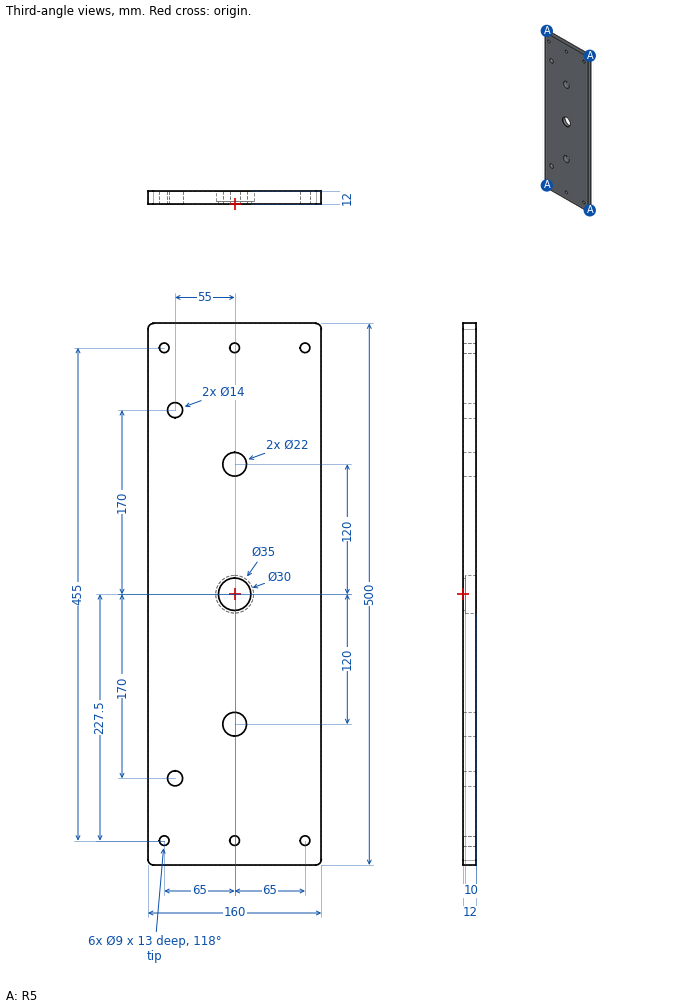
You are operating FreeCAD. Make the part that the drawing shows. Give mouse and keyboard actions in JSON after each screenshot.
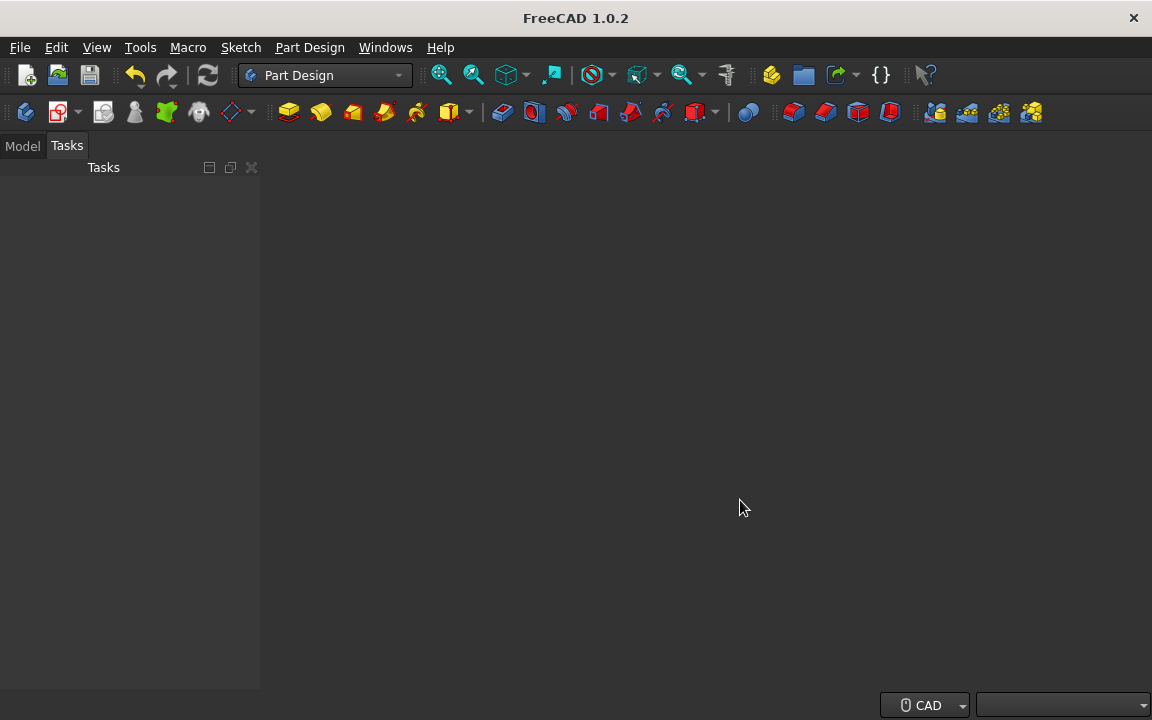
{"action": "left_click", "coordinate": [26, 76]}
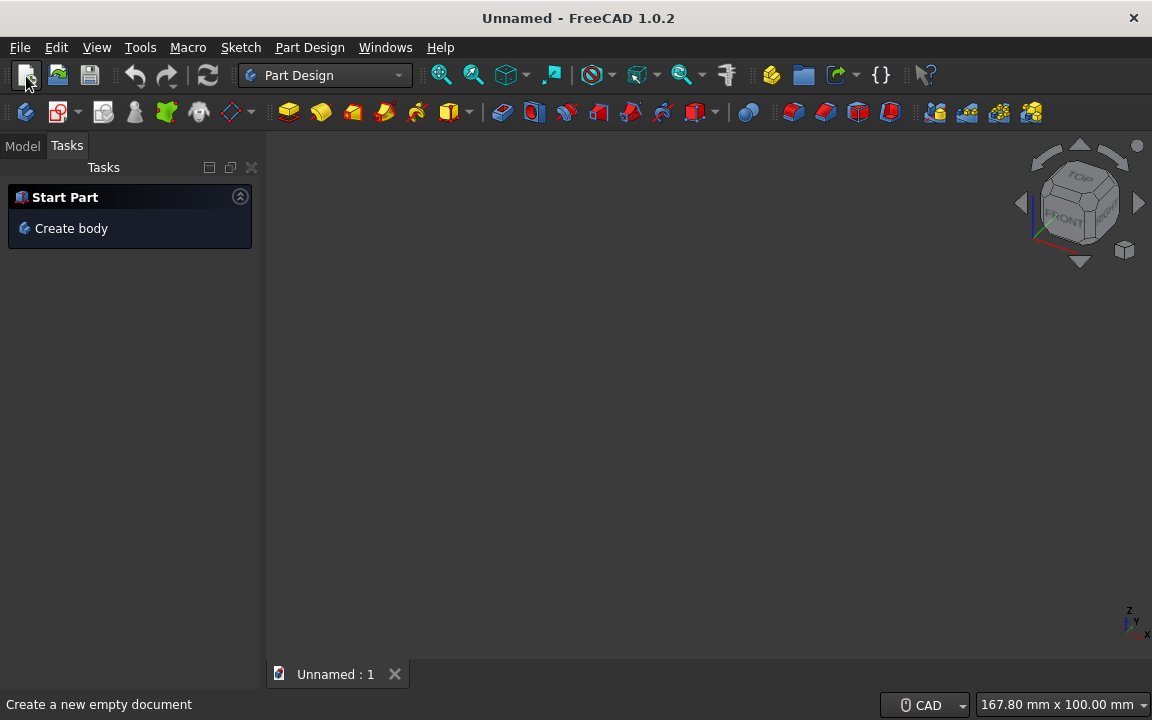
{"action": "left_click", "coordinate": [58, 112]}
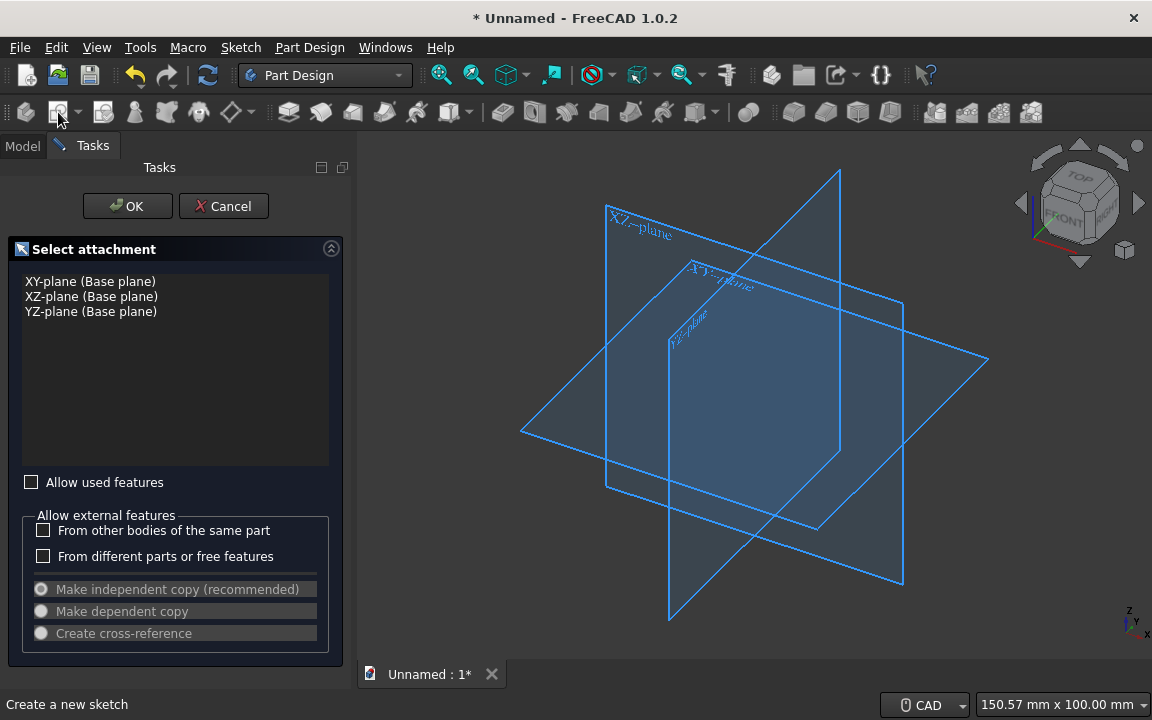
{"action": "left_click", "coordinate": [82, 296]}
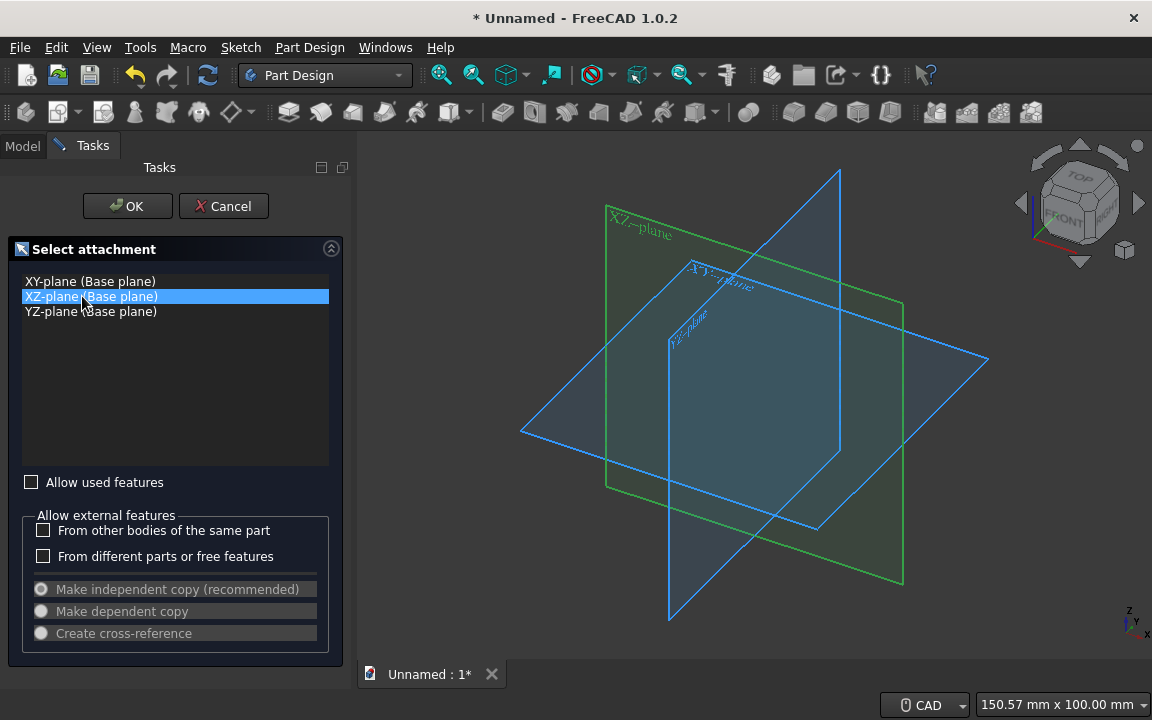
{"action": "left_click", "coordinate": [128, 206]}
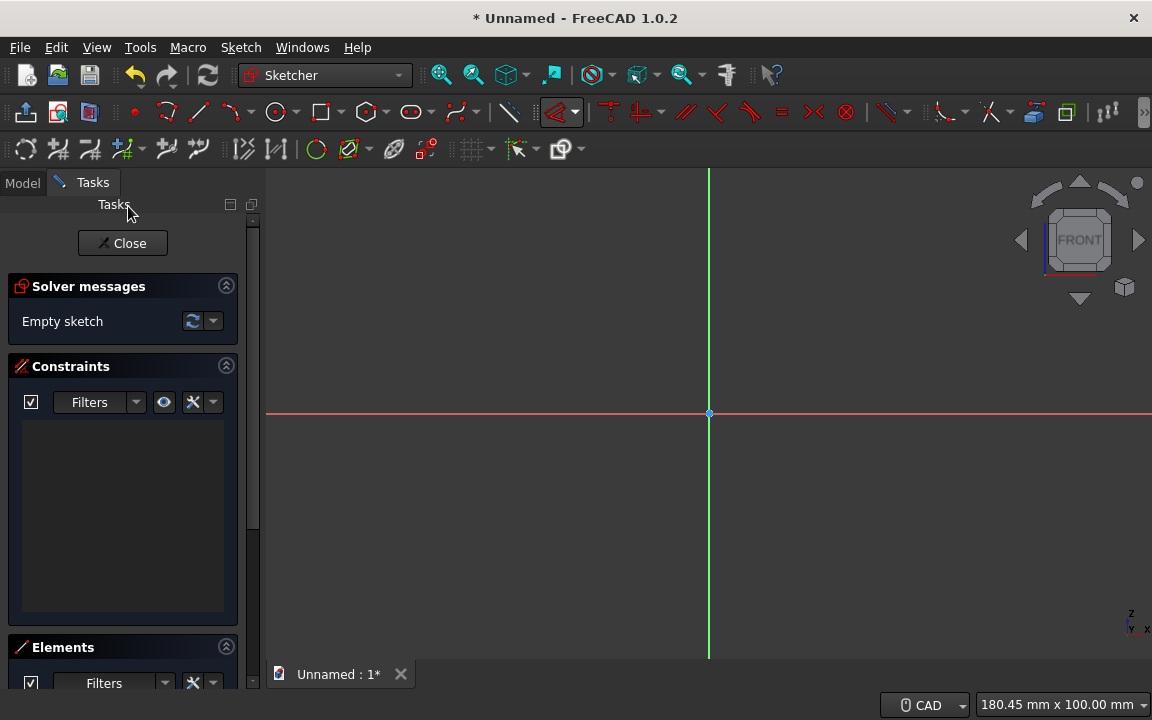
{"action": "scroll", "coordinate": [630, 414], "scroll_direction": "down", "scroll_amount": 10}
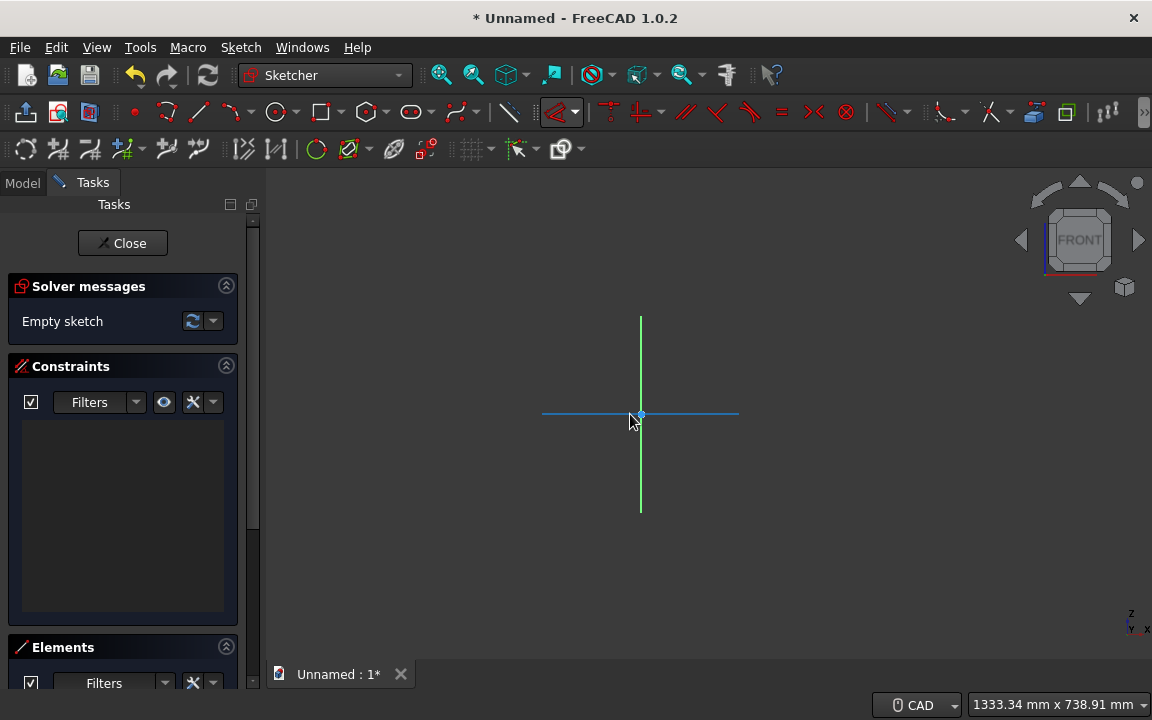
{"action": "key", "text": "g v"}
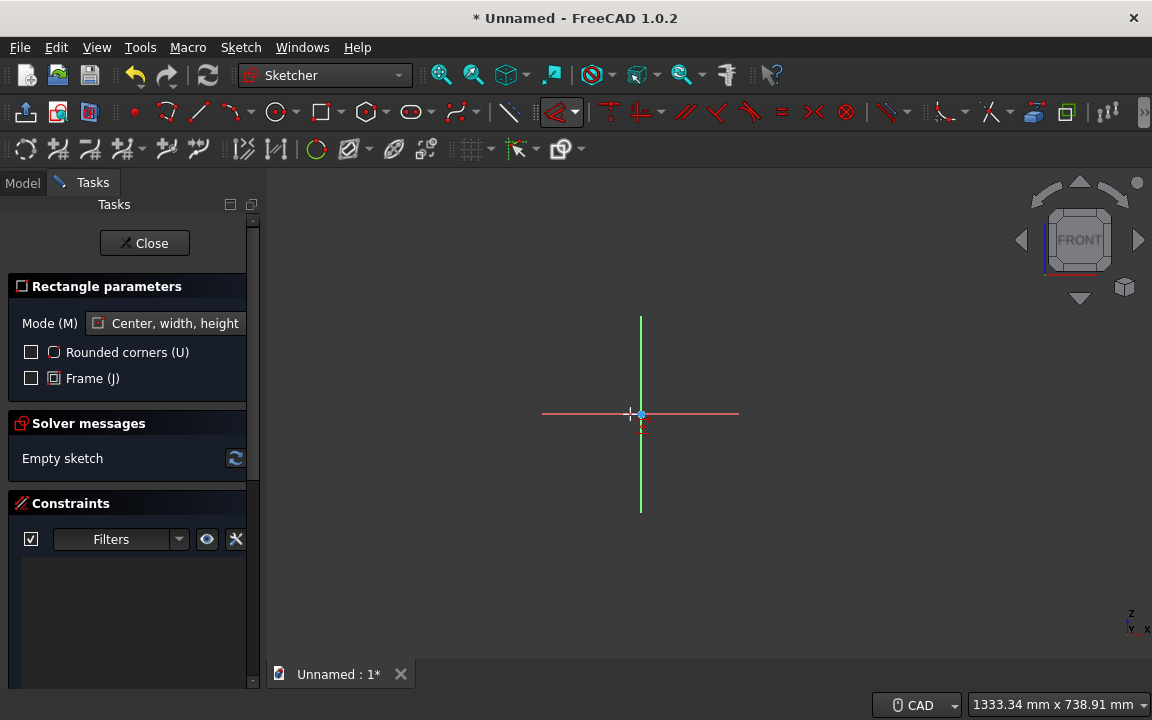
{"action": "left_click", "coordinate": [641, 414]}
{"action": "left_click", "coordinate": [694, 248]}
{"action": "key", "text": "Escape"}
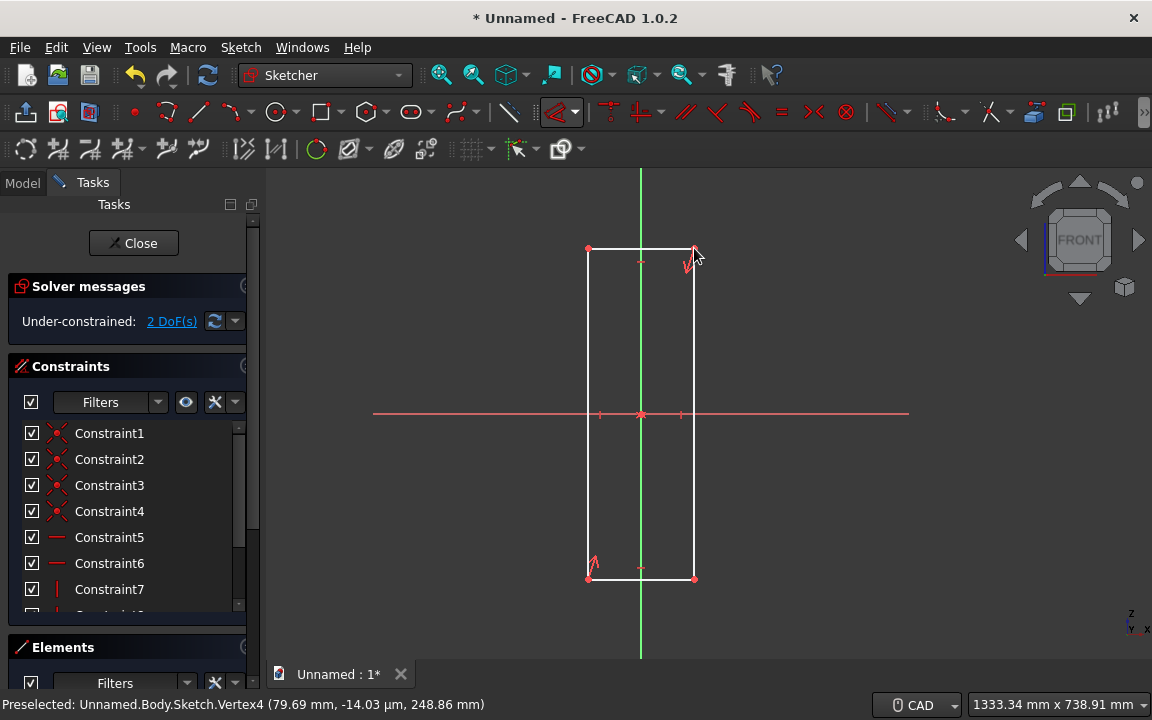
{"action": "left_click", "coordinate": [620, 580]}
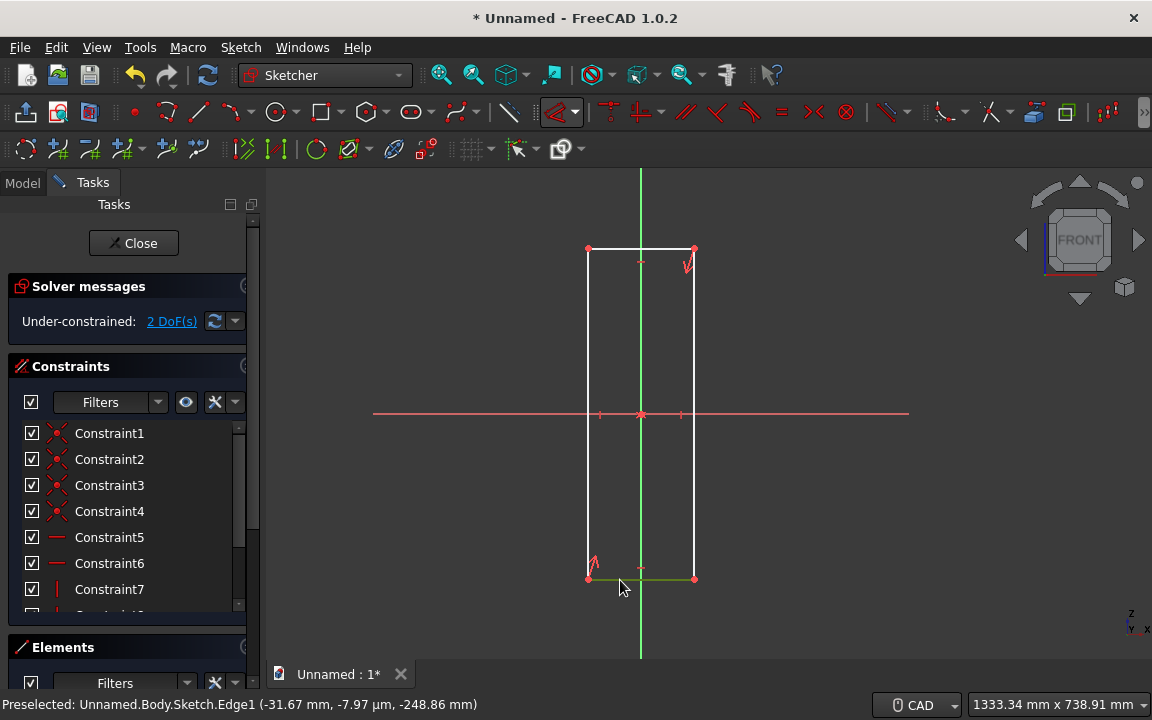
{"action": "key", "text": "l"}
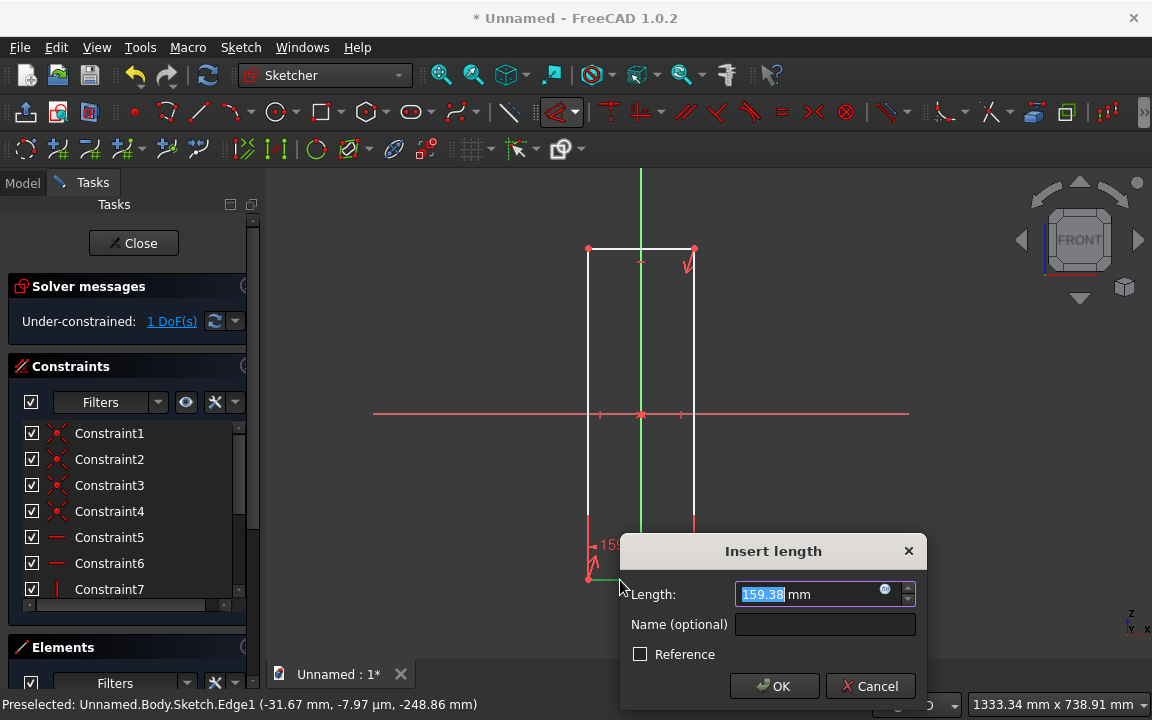
{"action": "type", "text": "160"}
{"action": "key", "text": "Return"}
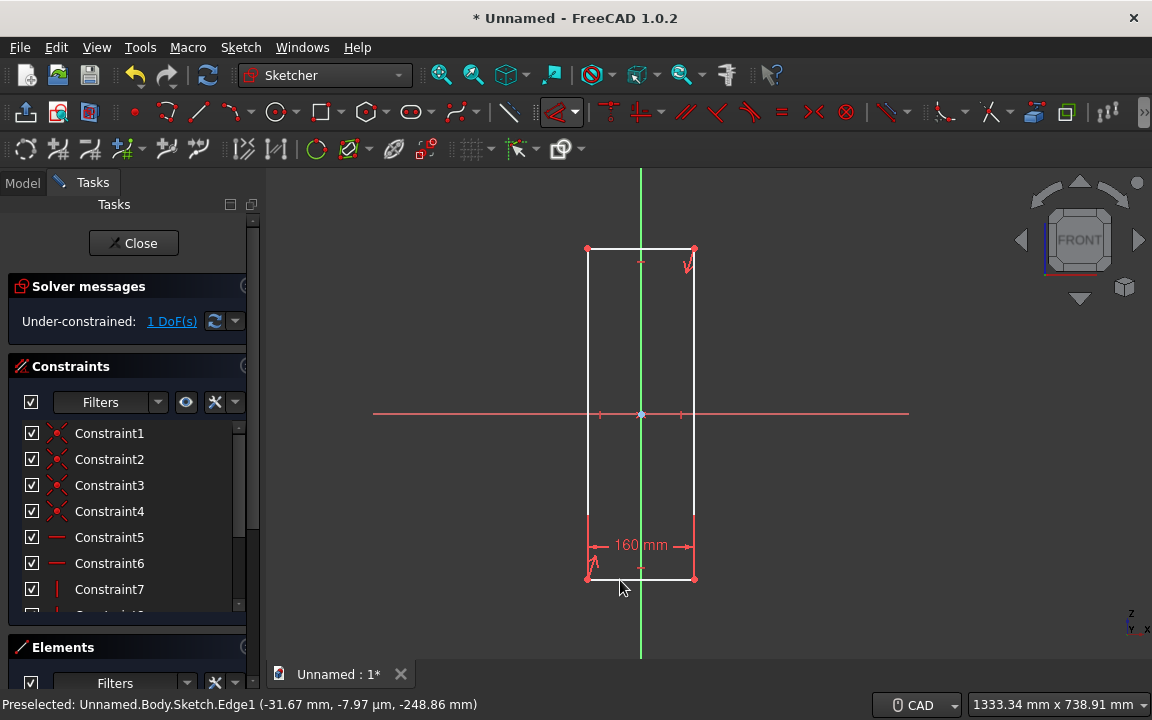
{"action": "left_click", "coordinate": [694, 481]}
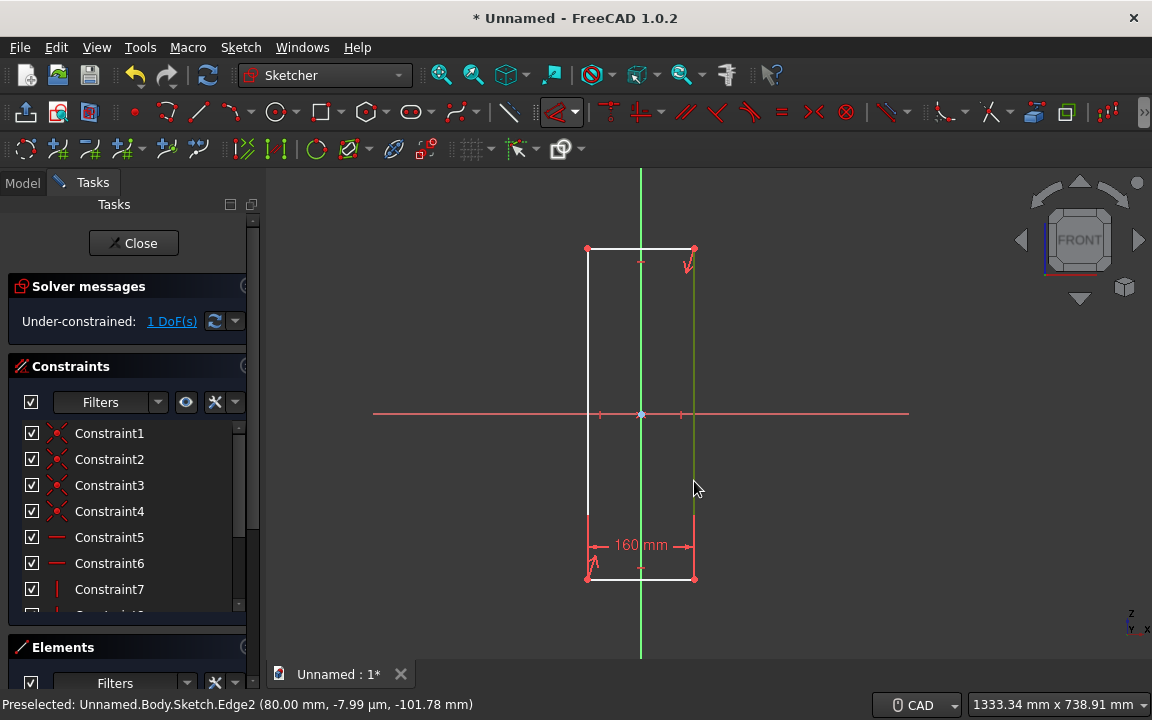
{"action": "key", "text": "i"}